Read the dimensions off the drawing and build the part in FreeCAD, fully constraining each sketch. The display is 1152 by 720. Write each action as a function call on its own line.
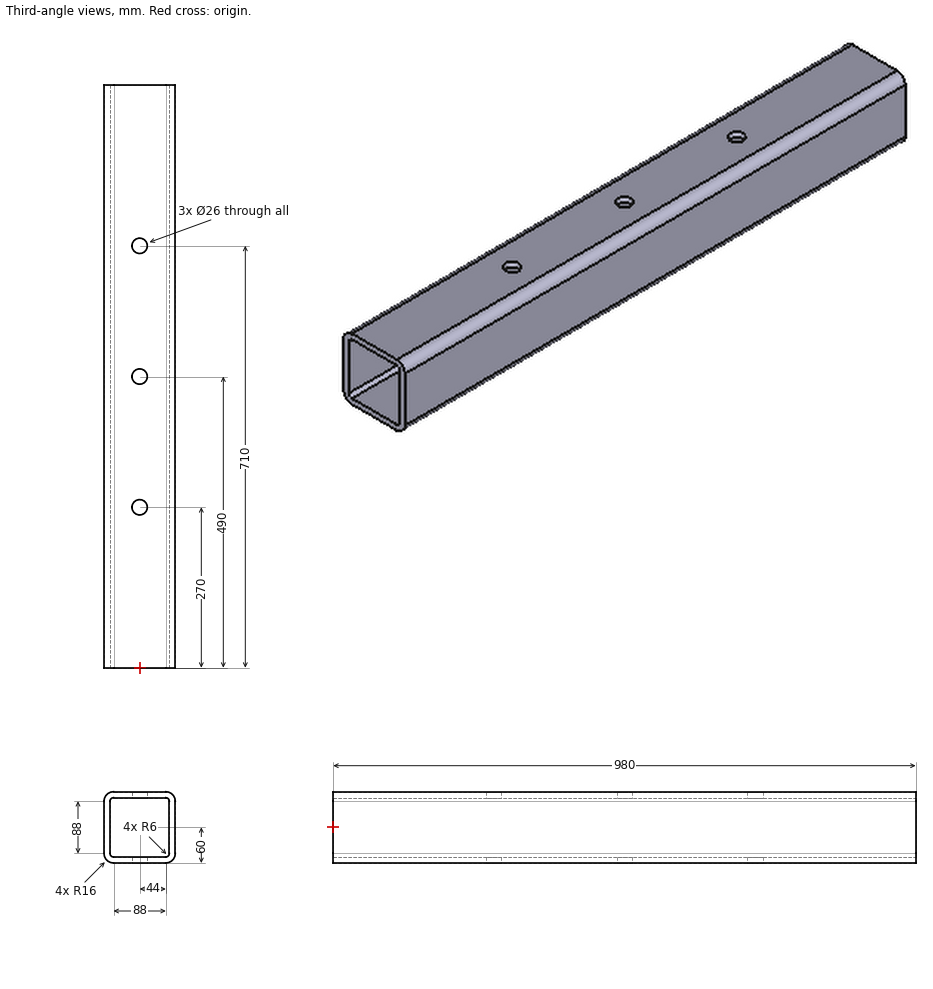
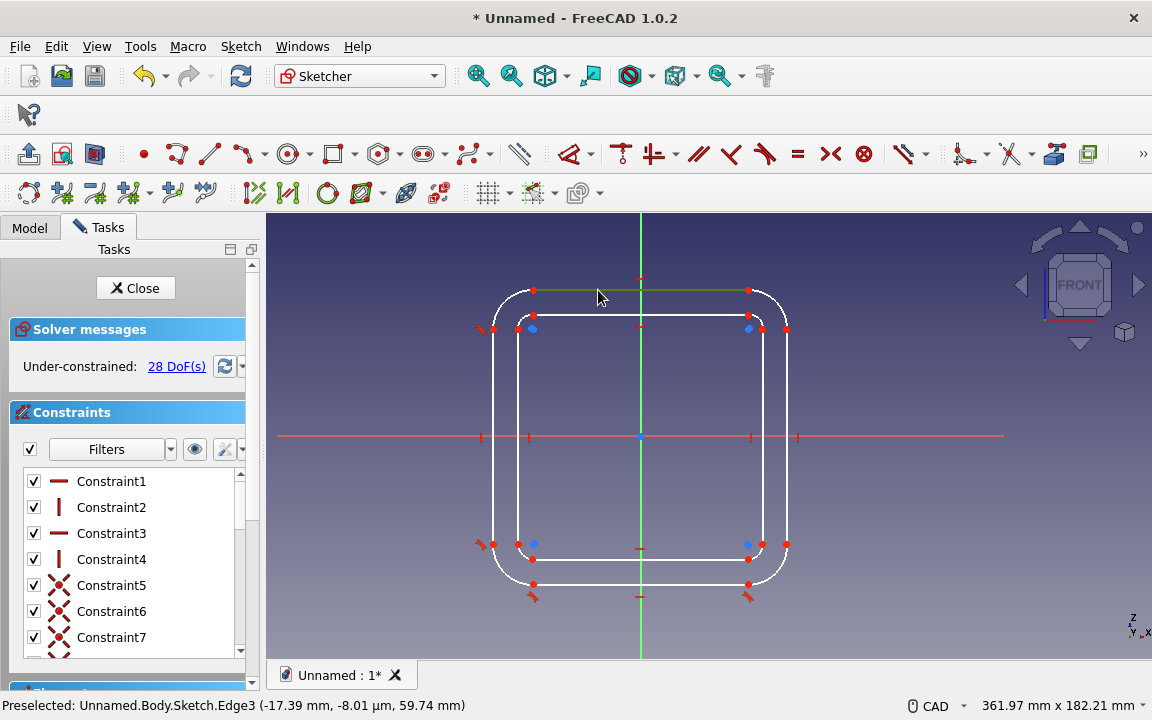
click(515, 294)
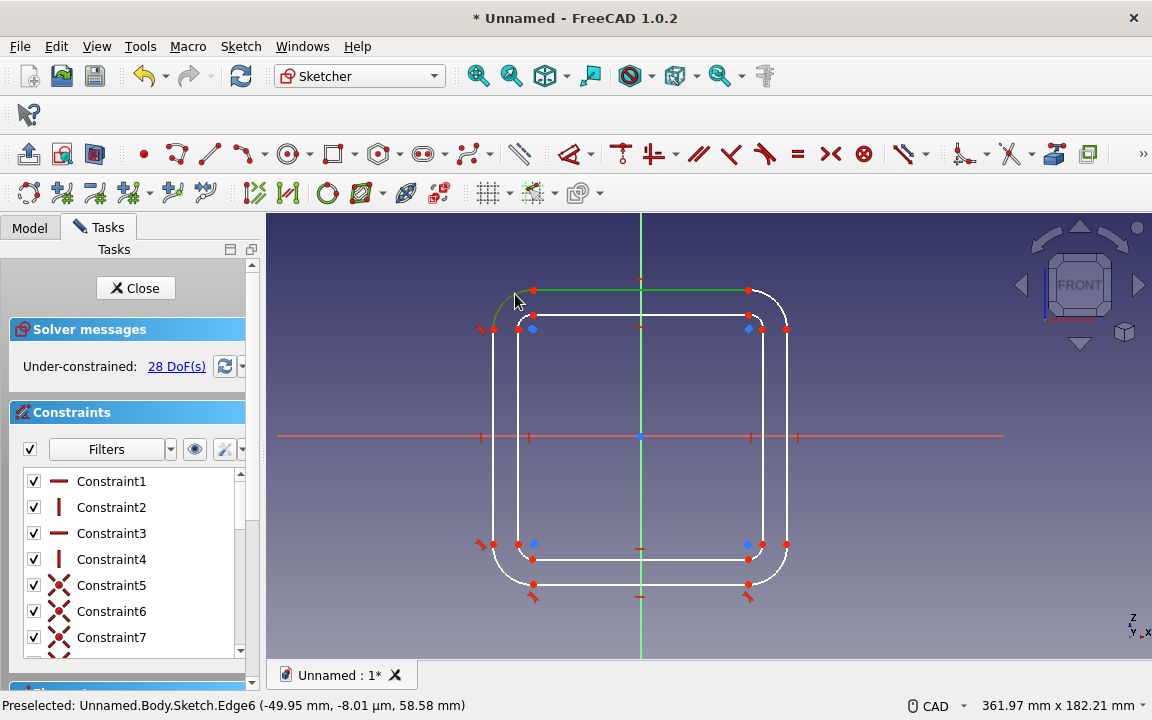
click(765, 154)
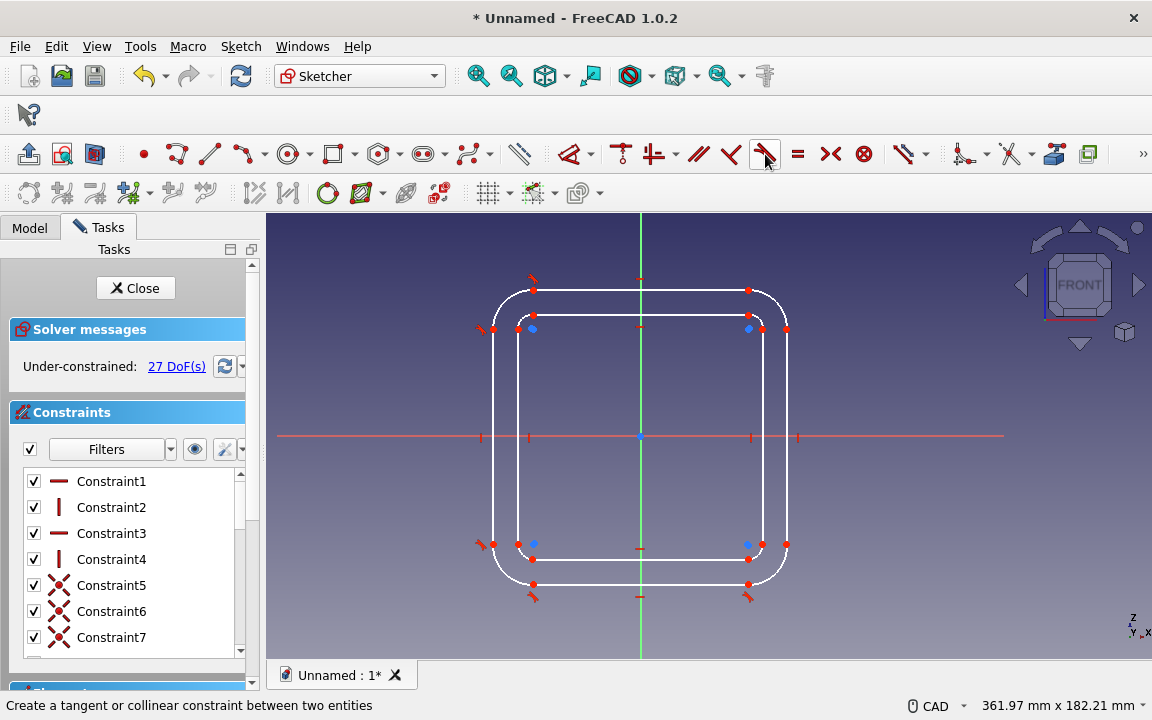
click(598, 290)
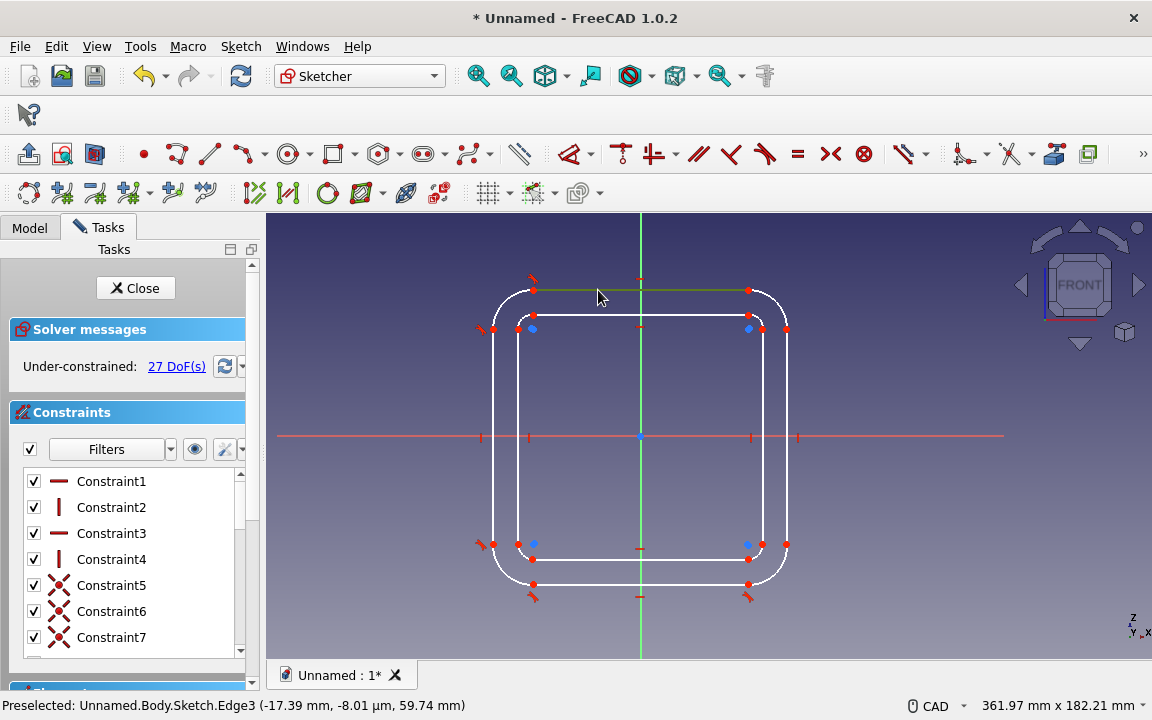
click(783, 312)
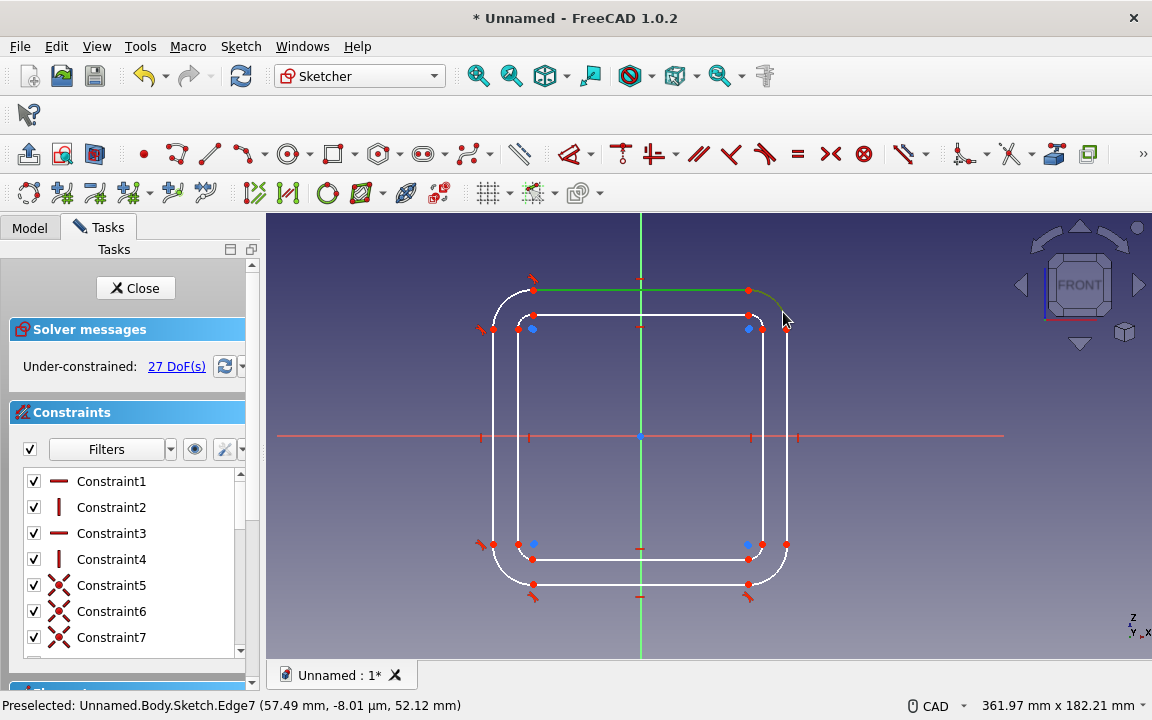
click(765, 154)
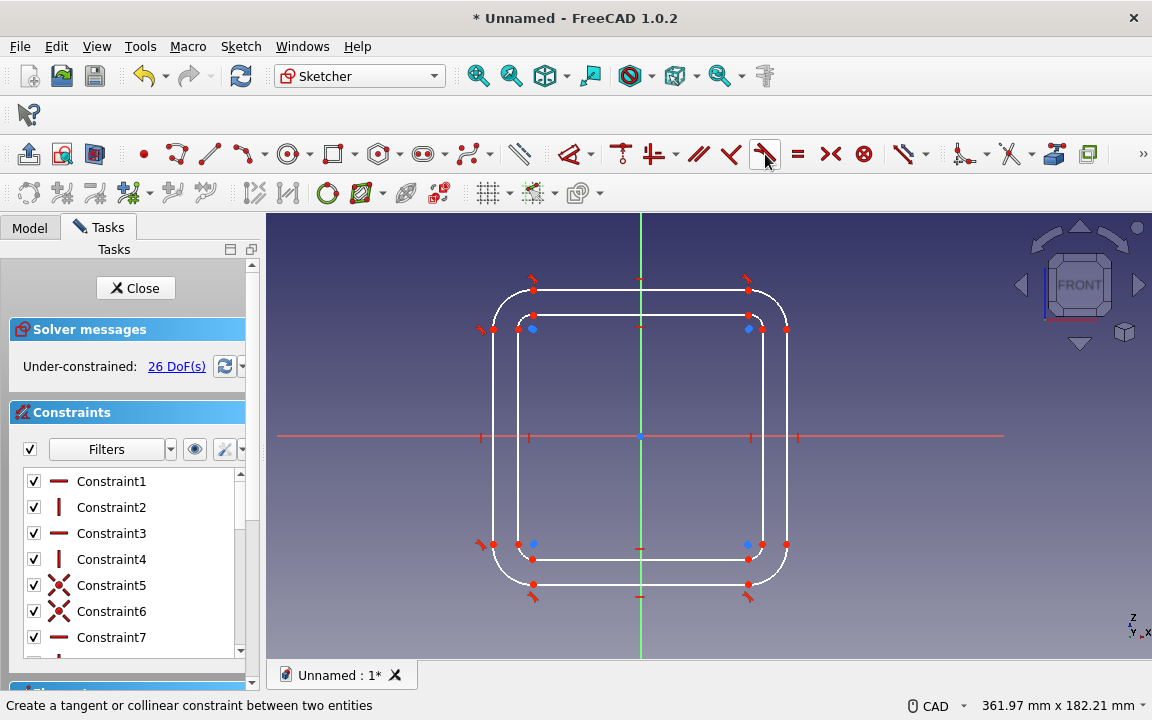
click(787, 395)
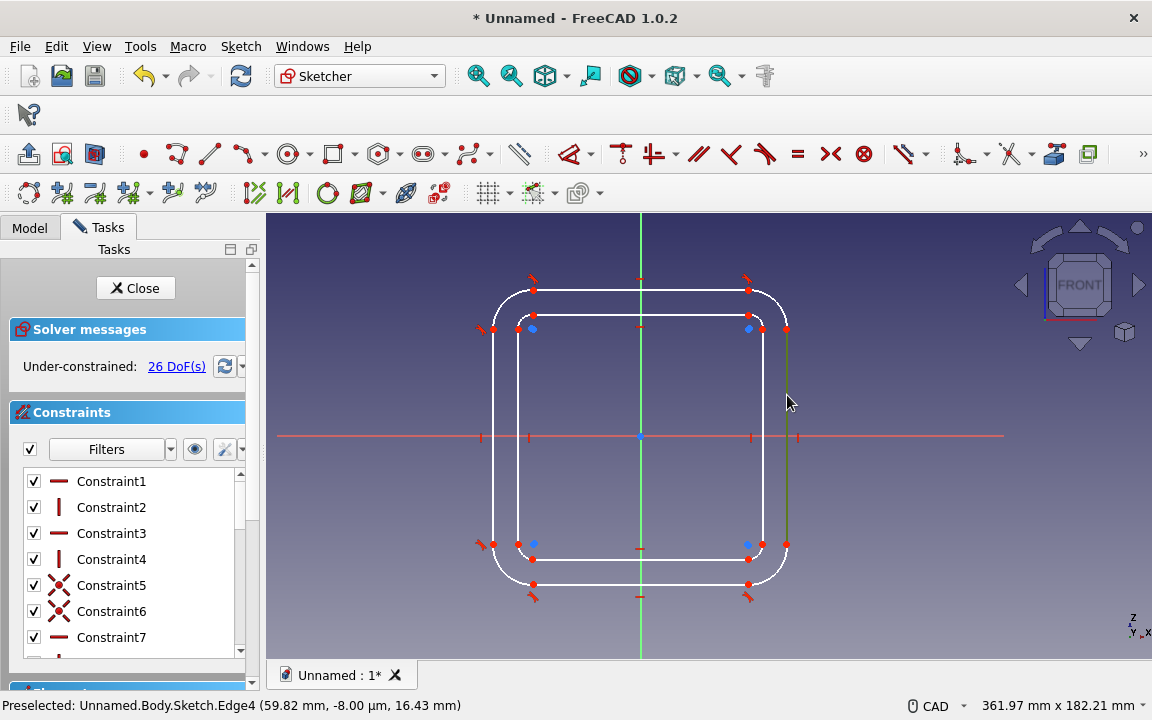
click(783, 312)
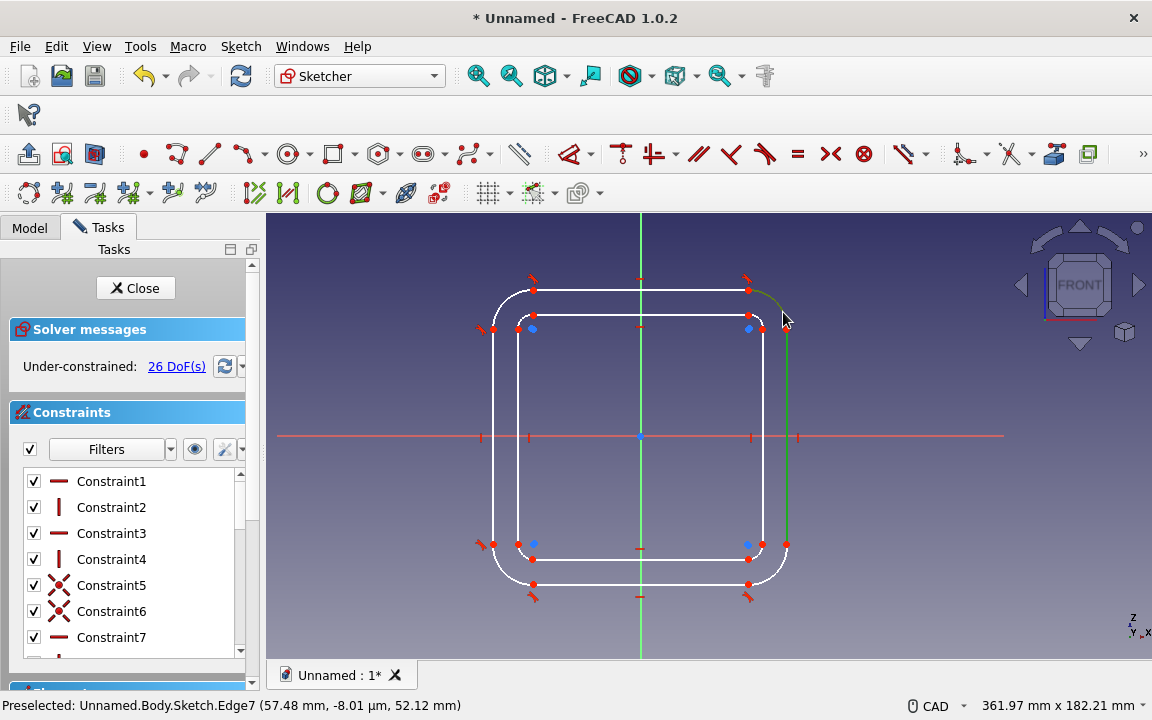
click(765, 154)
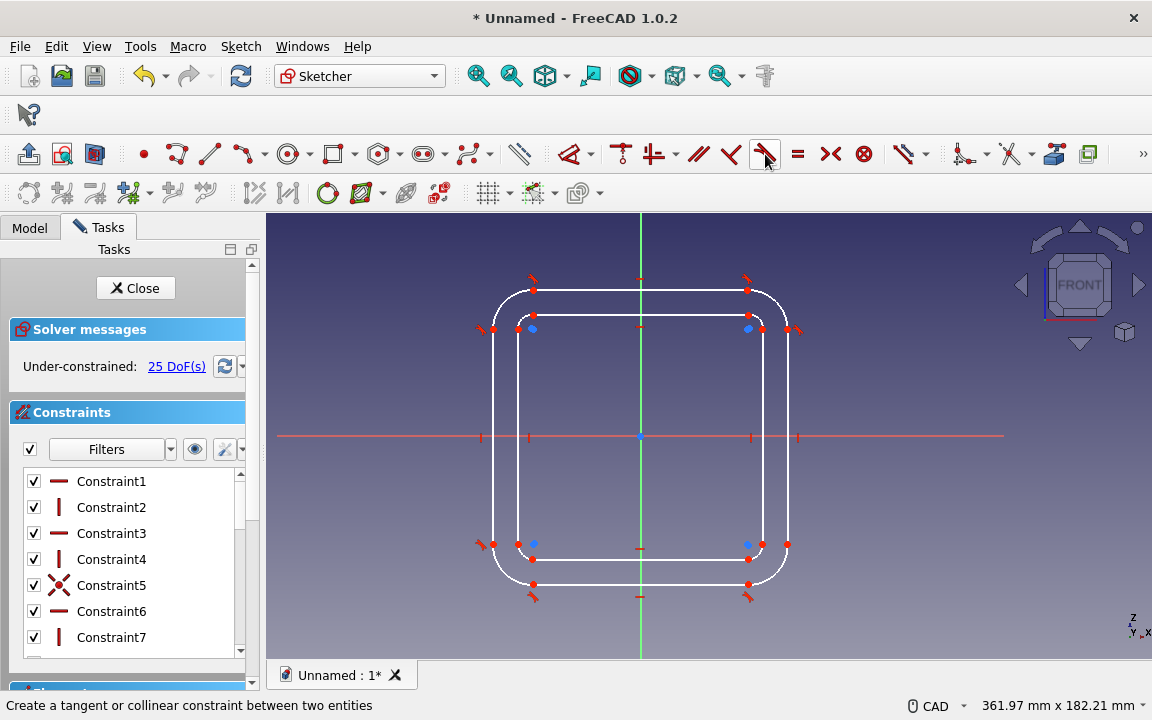
click(788, 394)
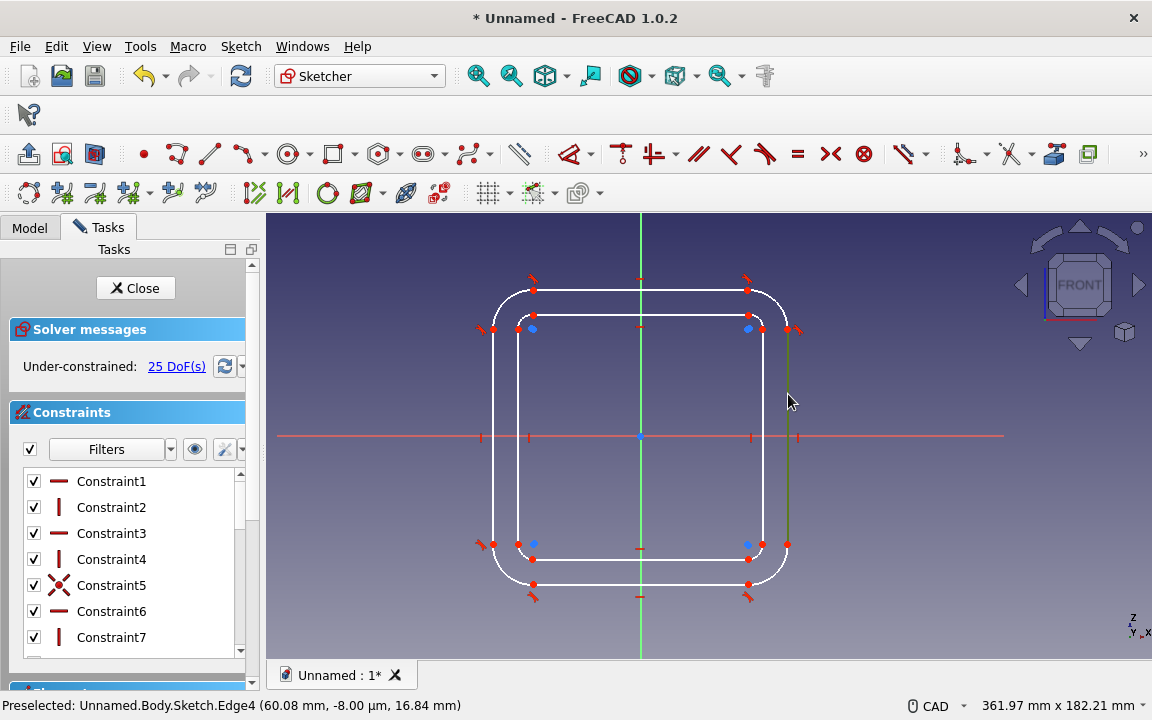
click(766, 581)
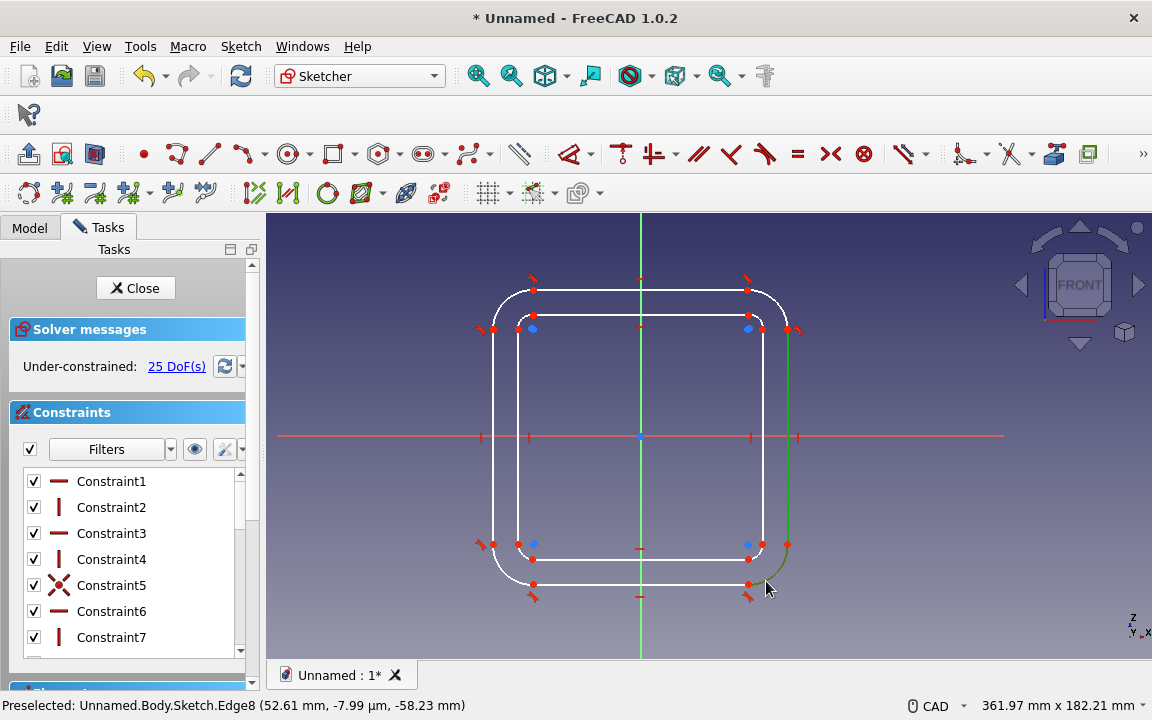
click(765, 154)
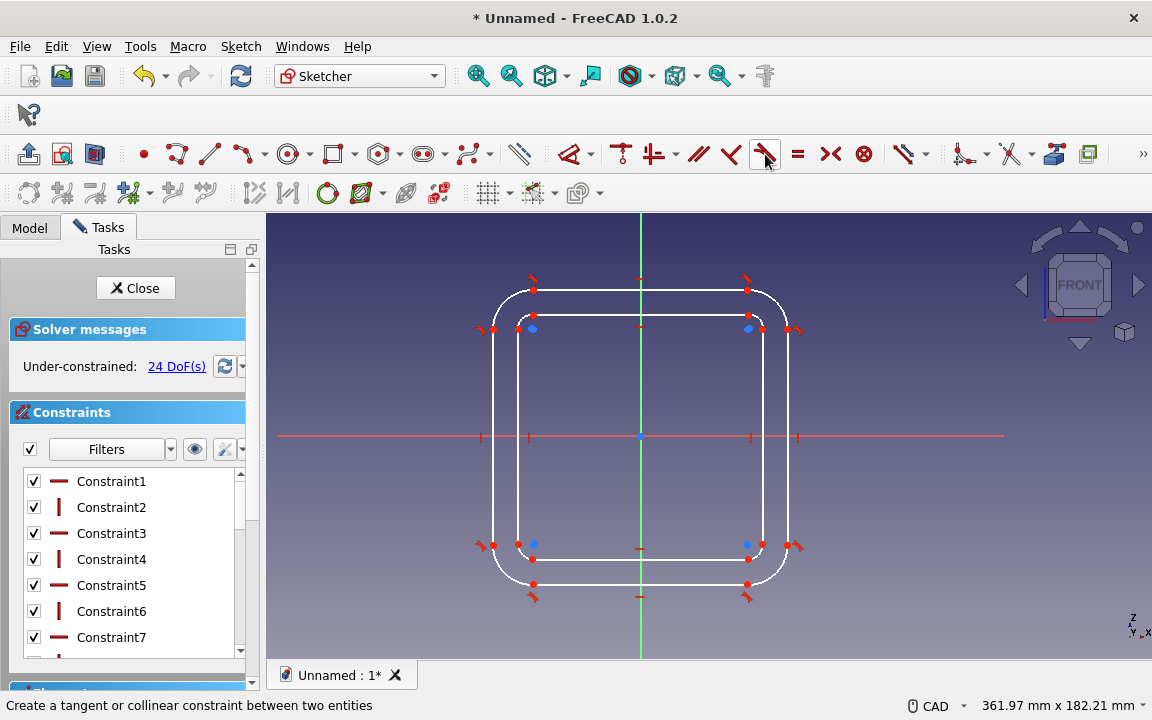
click(597, 560)